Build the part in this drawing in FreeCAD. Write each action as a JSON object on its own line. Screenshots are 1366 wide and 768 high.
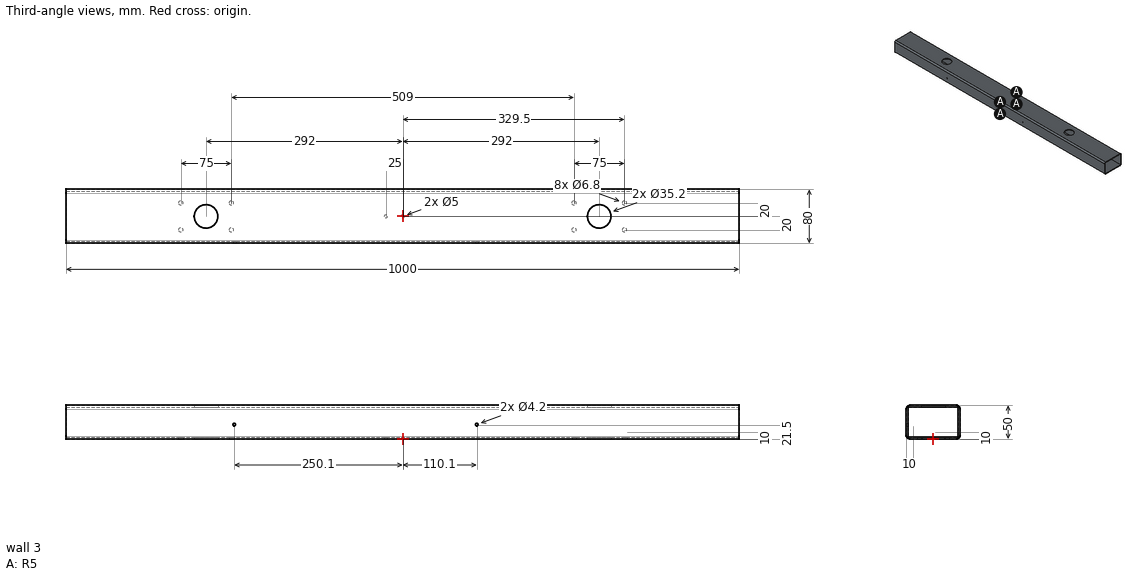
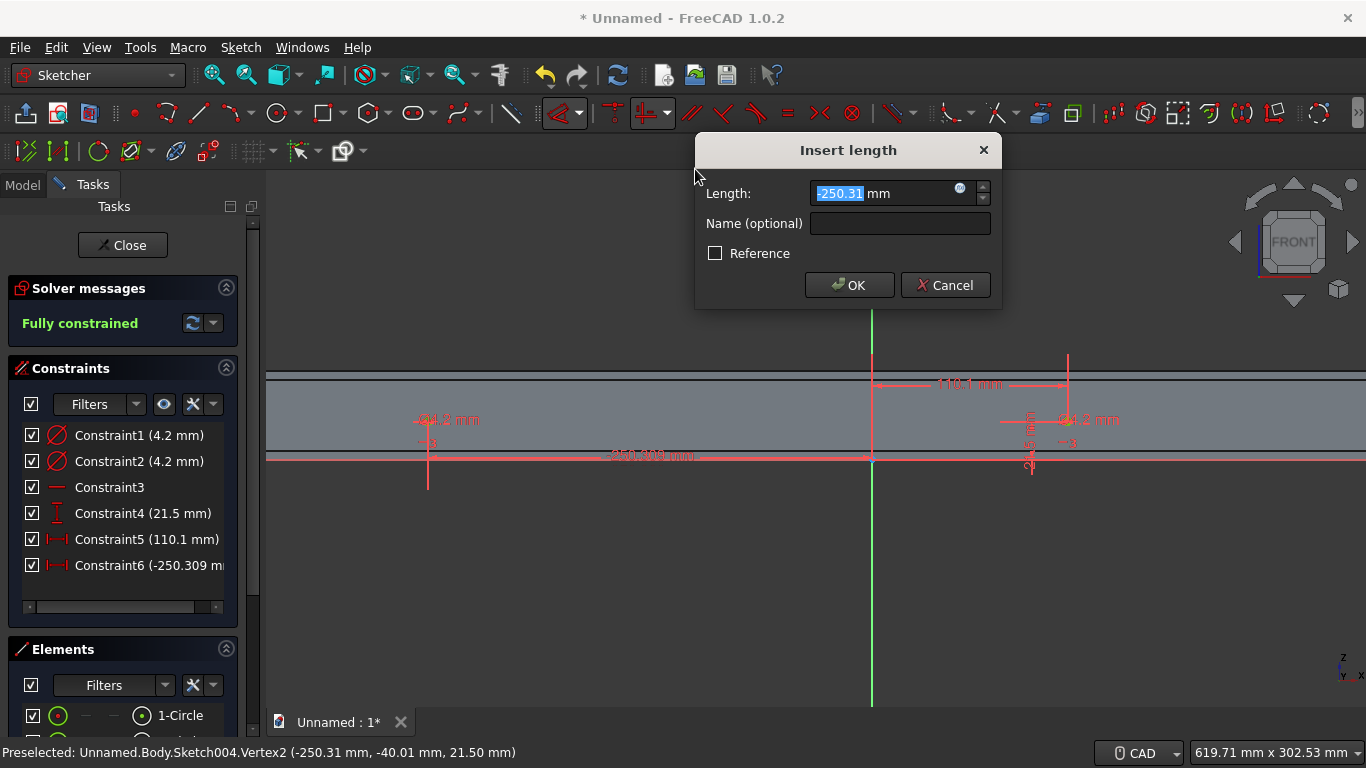
{"action": "type", "text": "-250.1"}
{"action": "key", "text": "Return"}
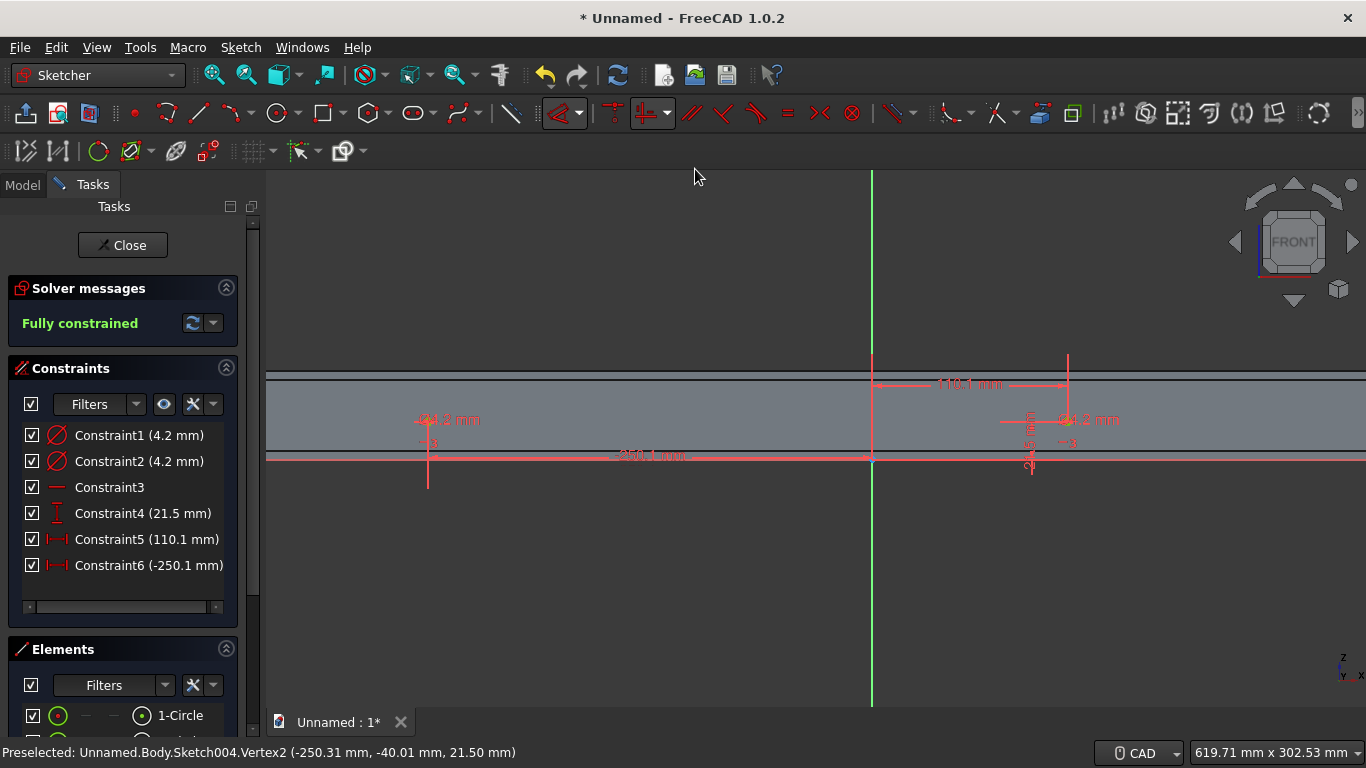
{"action": "left_click", "coordinate": [123, 245]}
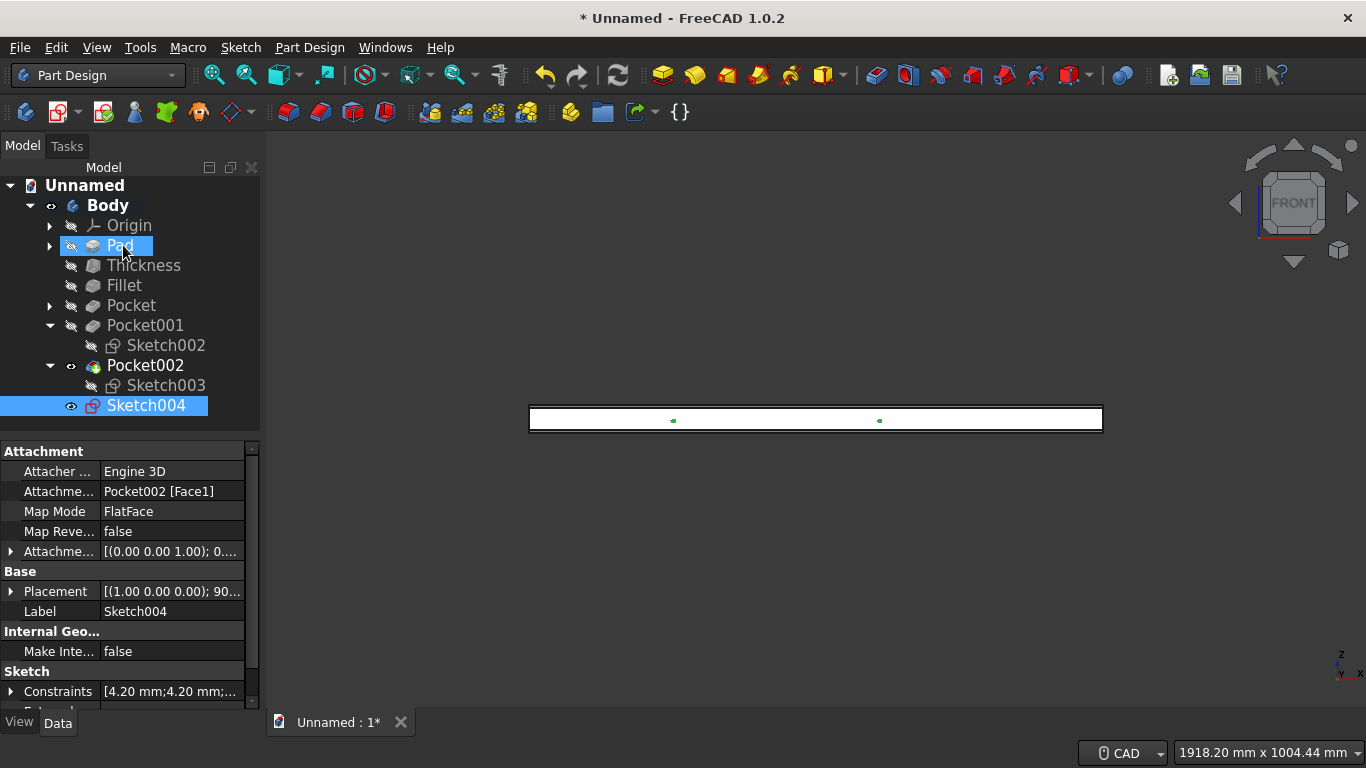
{"action": "left_click", "coordinate": [878, 76]}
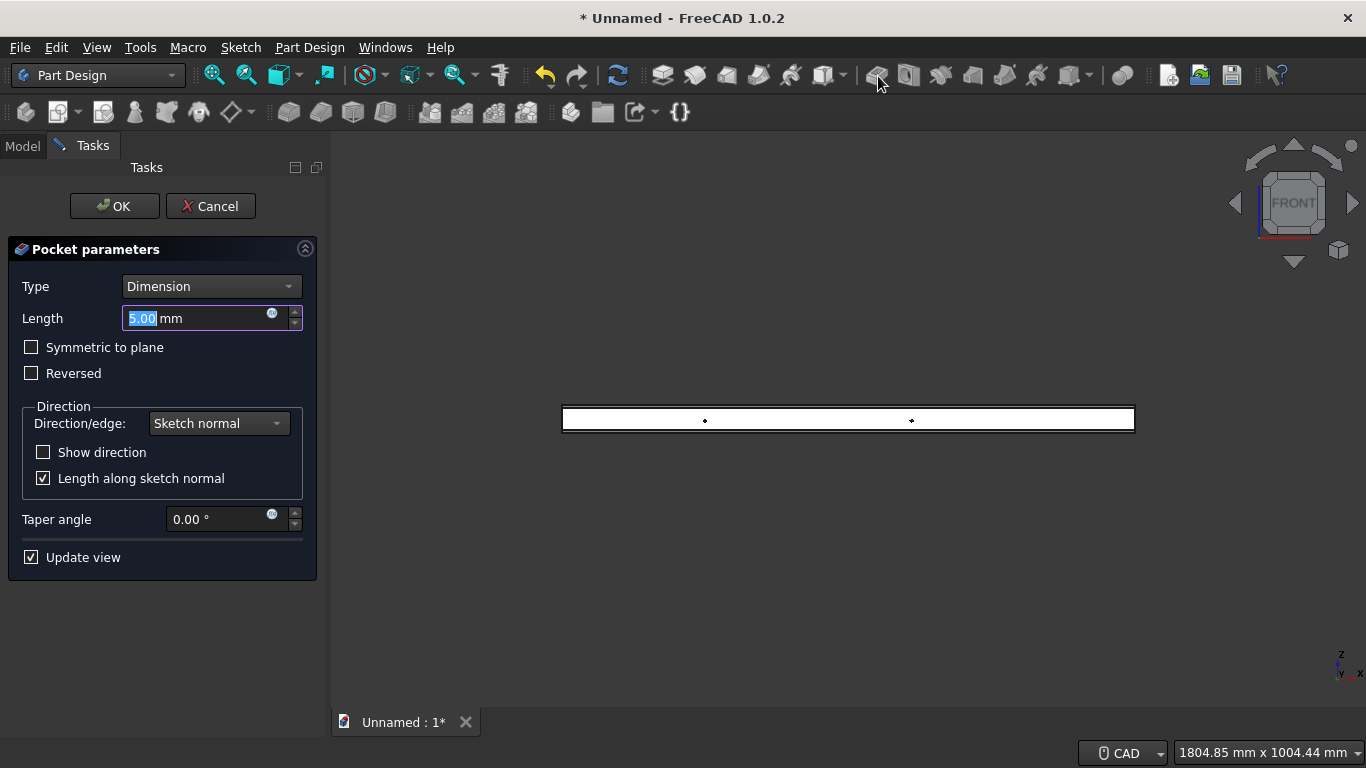
{"action": "type", "text": "10"}
{"action": "key", "text": "Tab"}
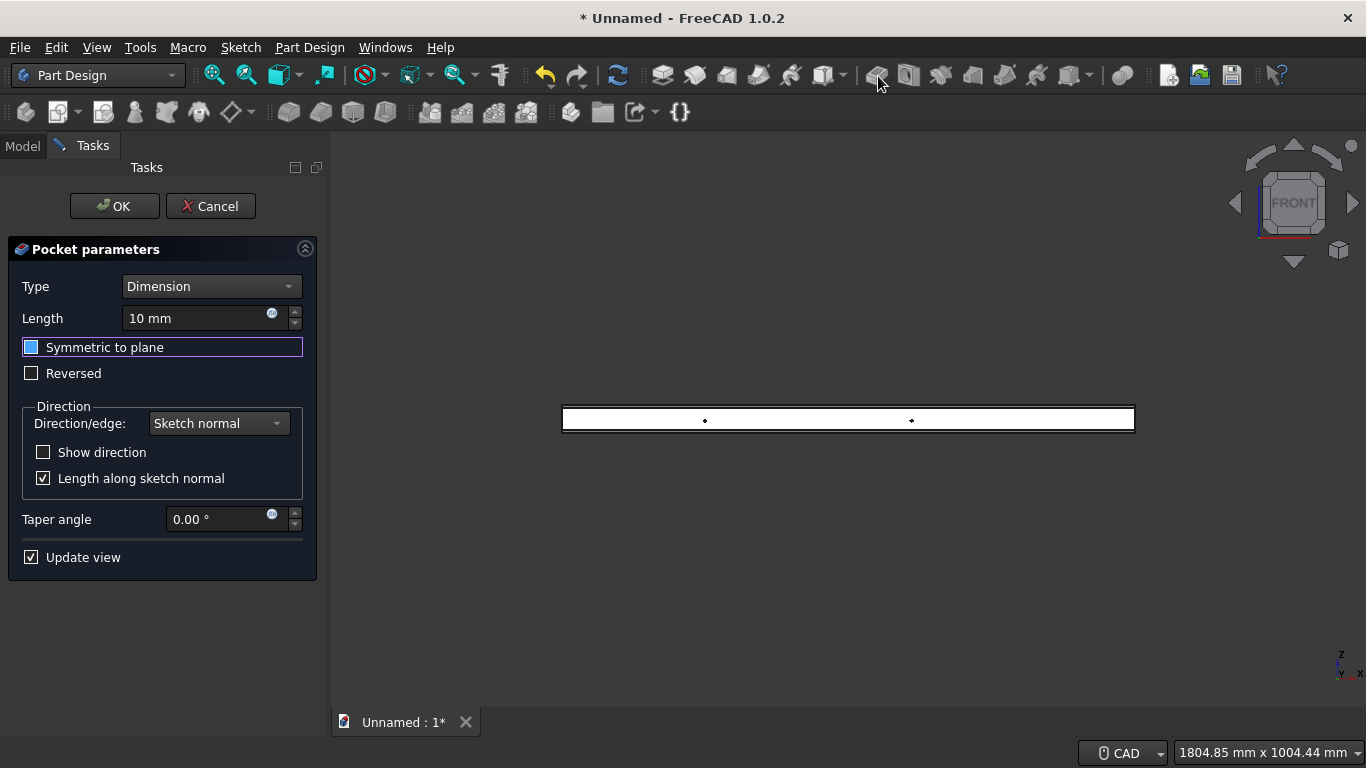
{"action": "left_click", "coordinate": [115, 206]}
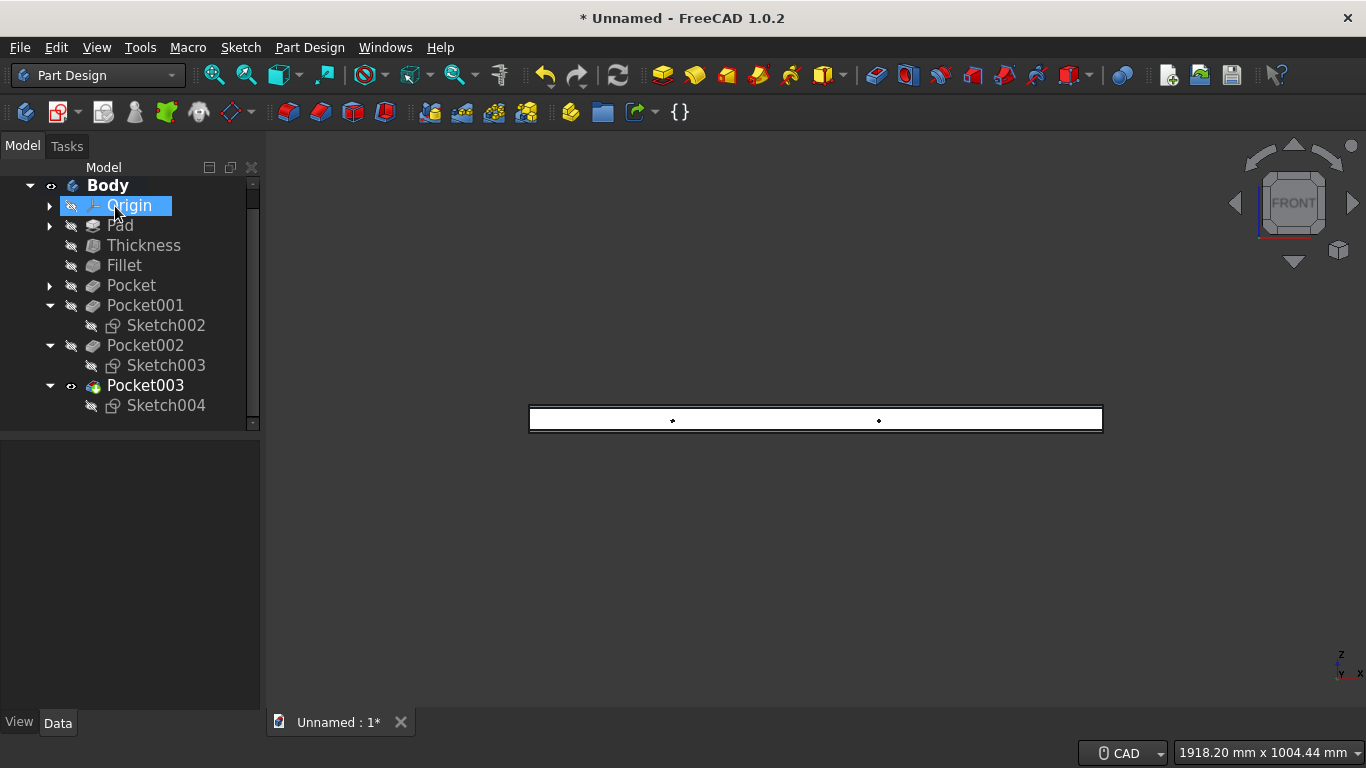
{"action": "key", "text": "0"}